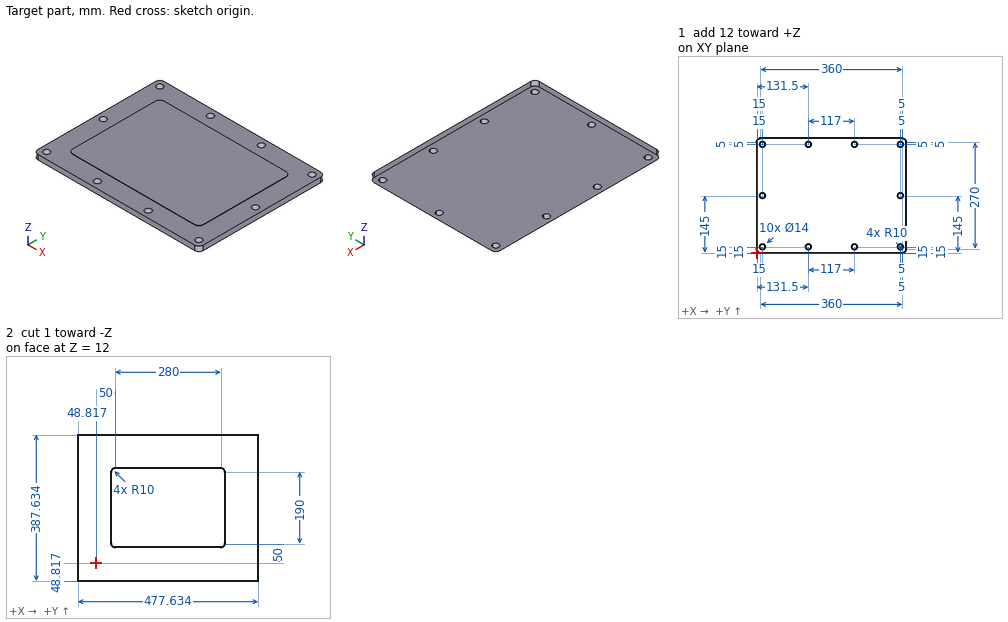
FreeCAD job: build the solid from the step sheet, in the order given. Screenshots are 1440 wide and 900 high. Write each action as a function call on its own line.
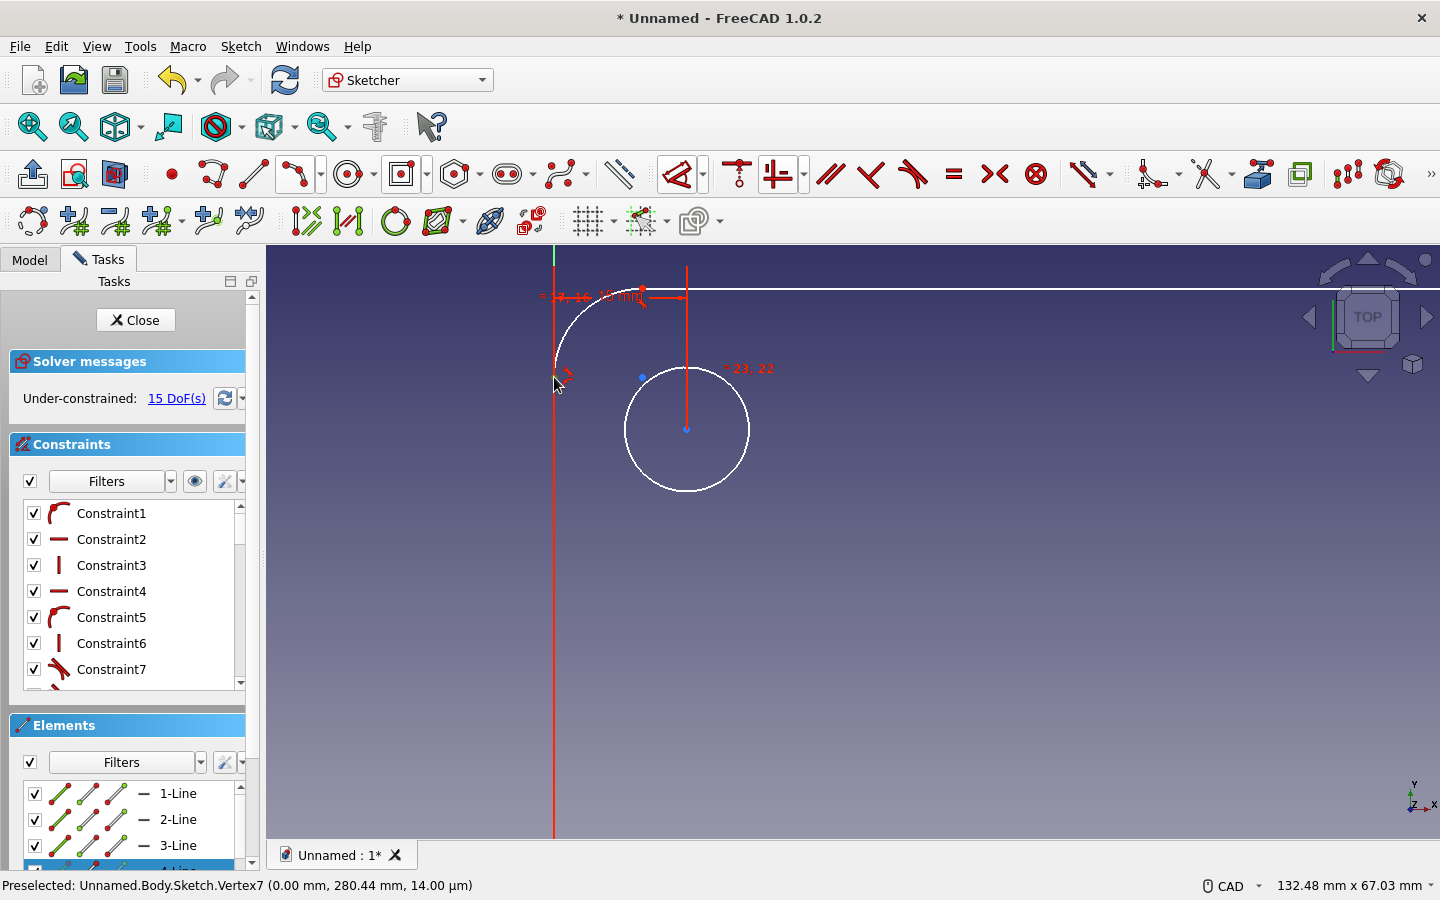
click(687, 429)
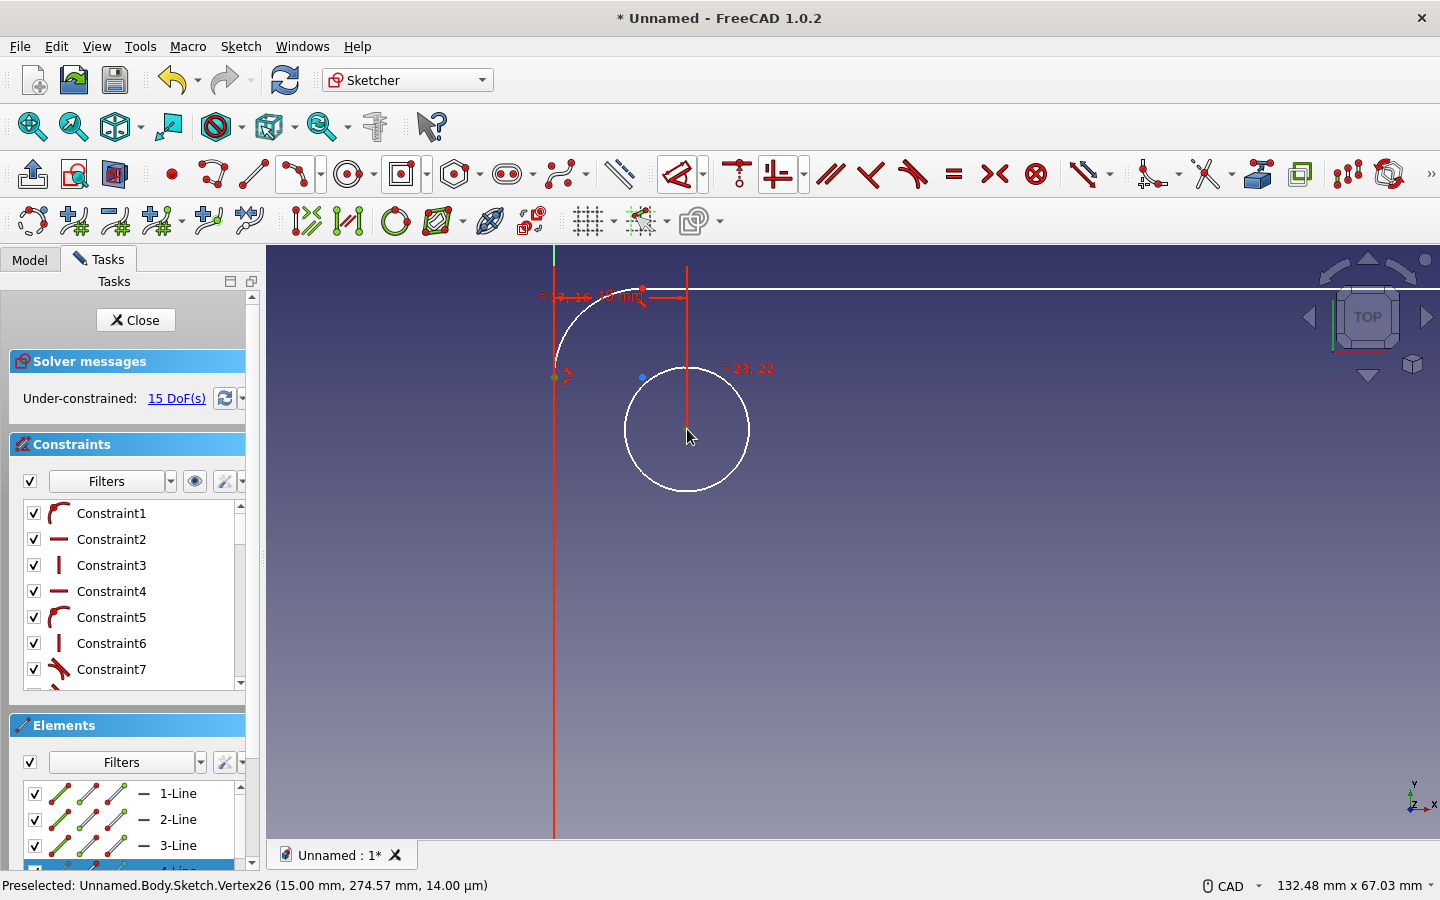
key(i)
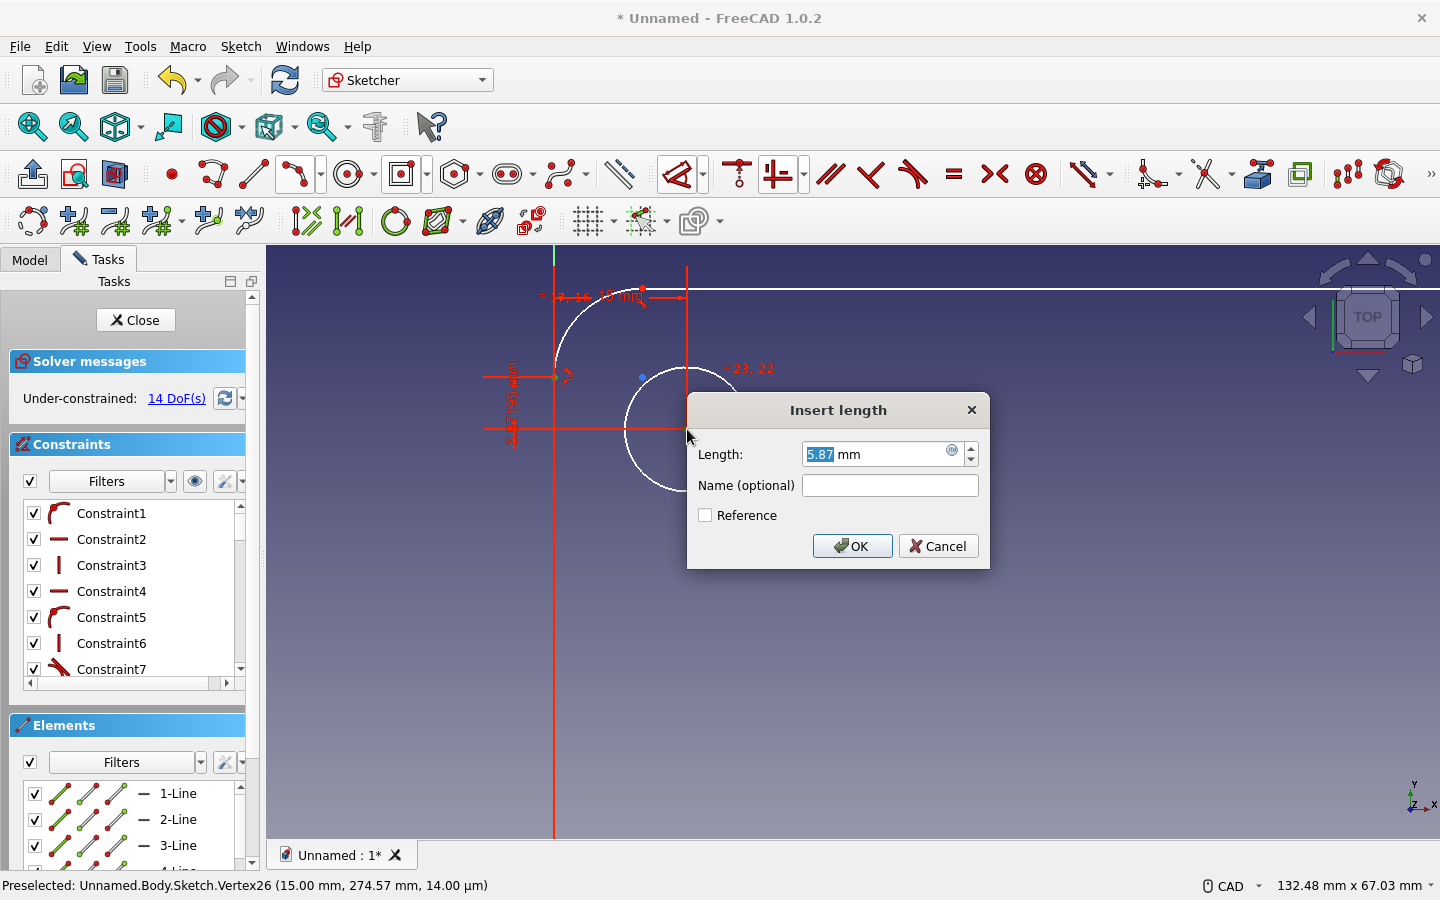
text(5)
key(Return)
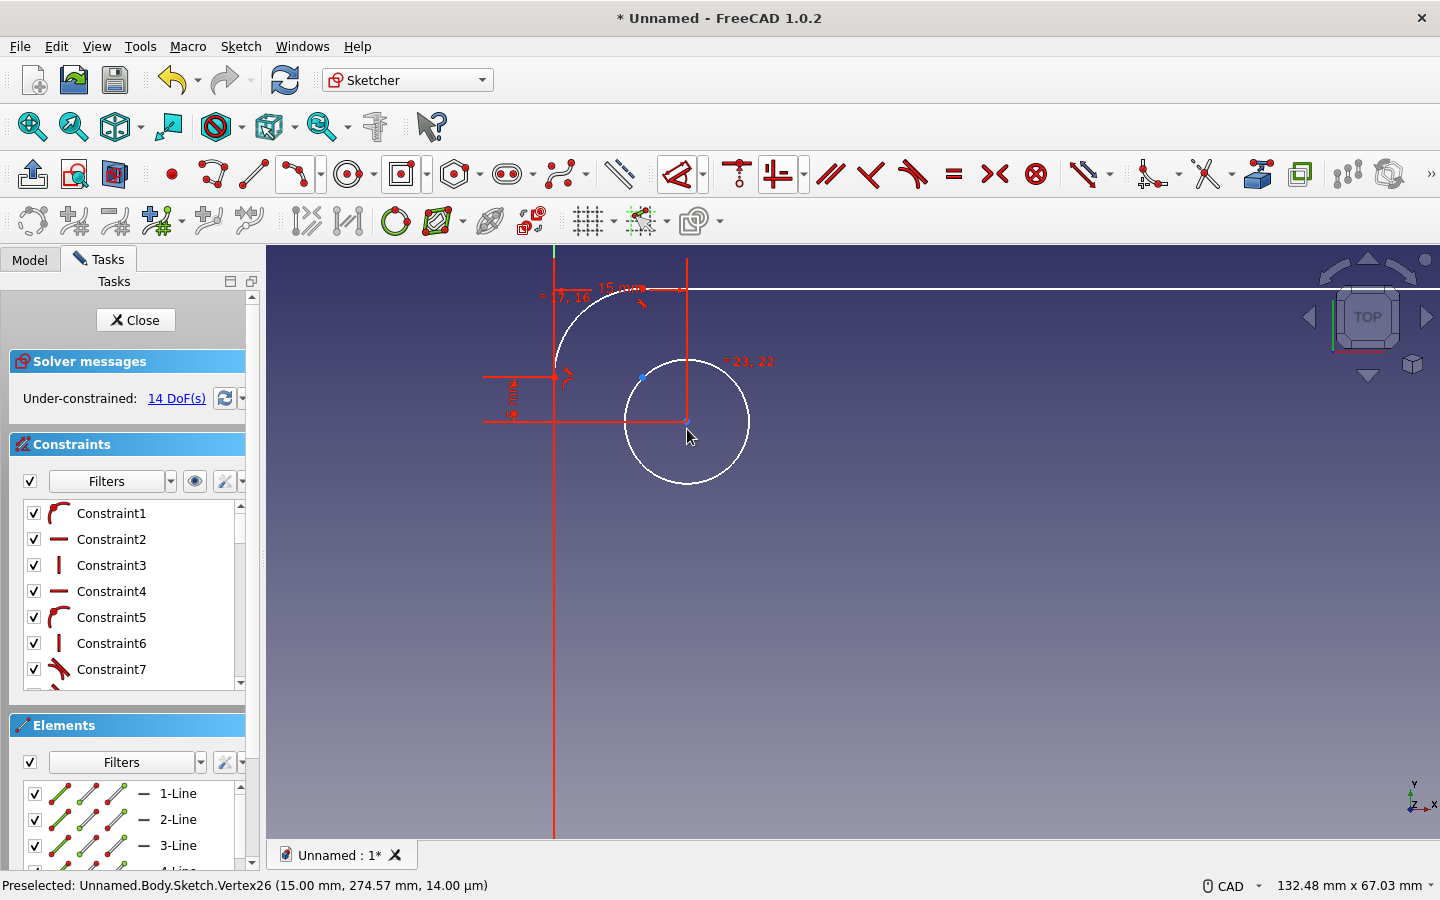
click(554, 377)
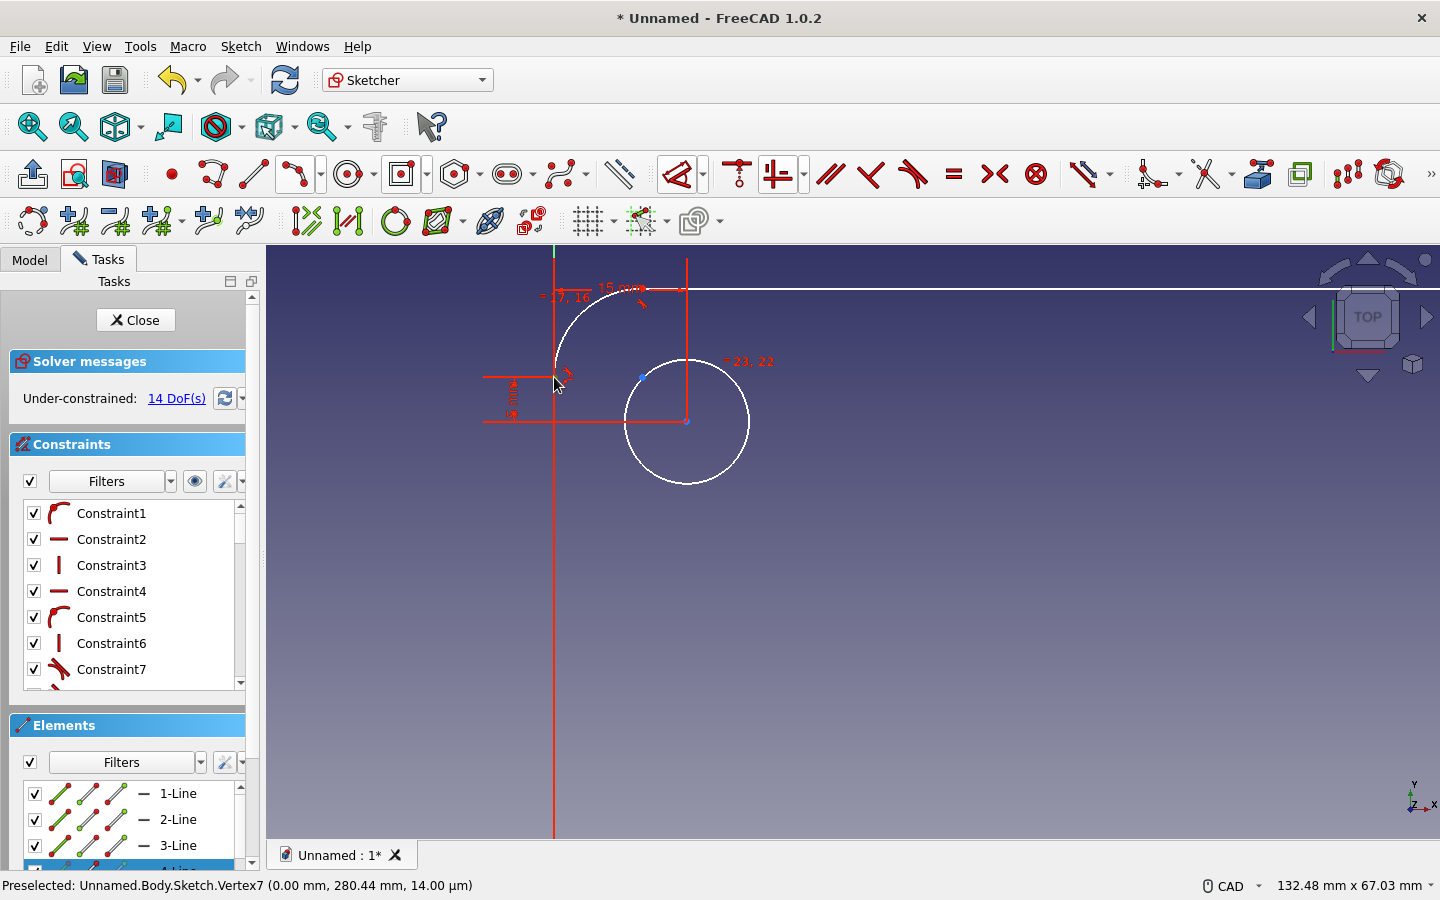
scroll(557, 380, down, 10)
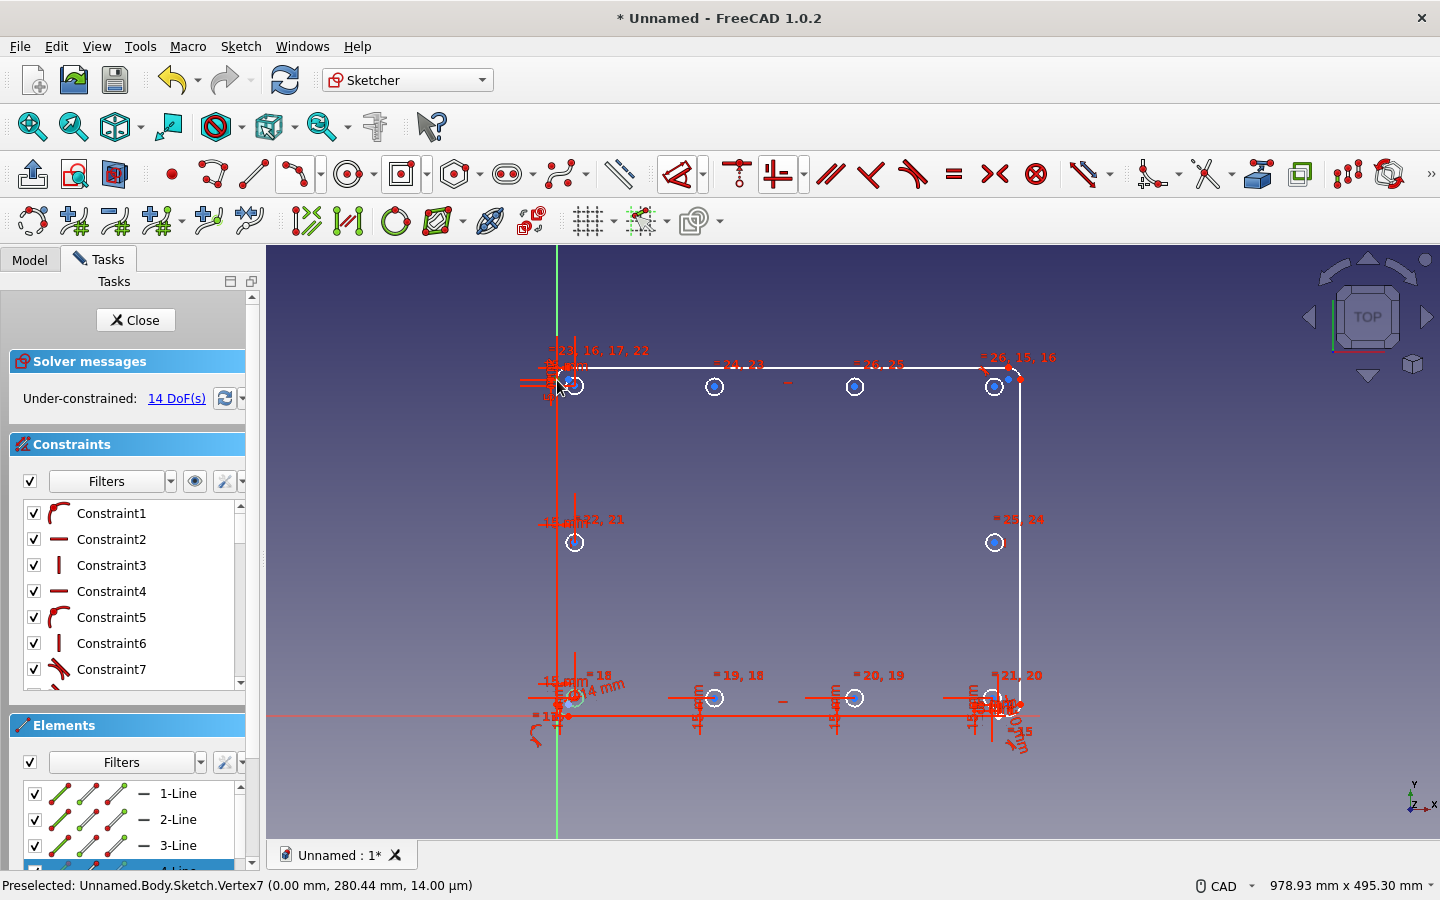
scroll(715, 387, up, 10)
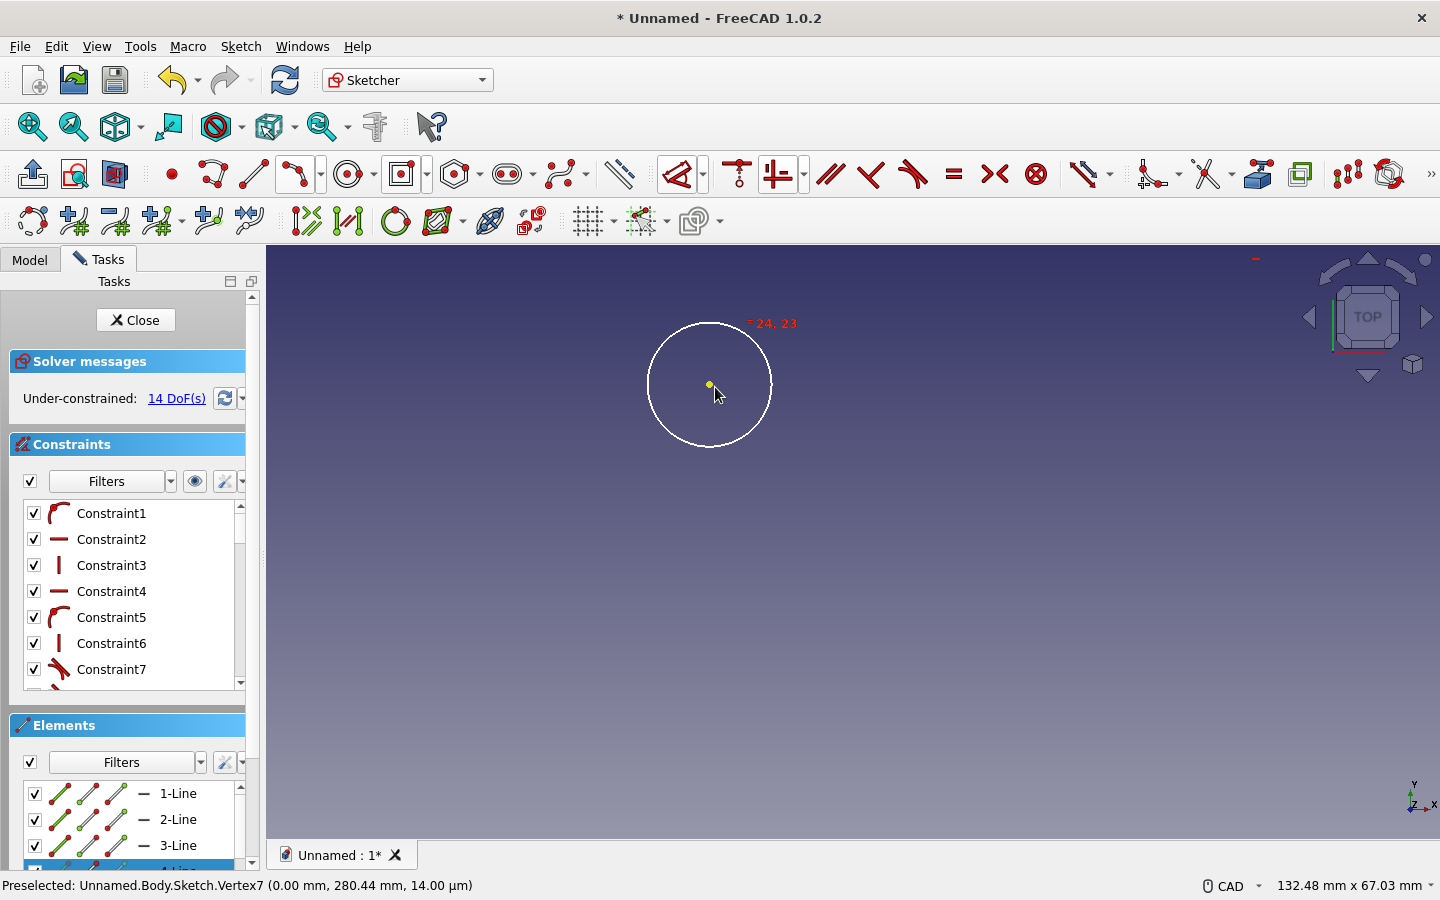
click(710, 385)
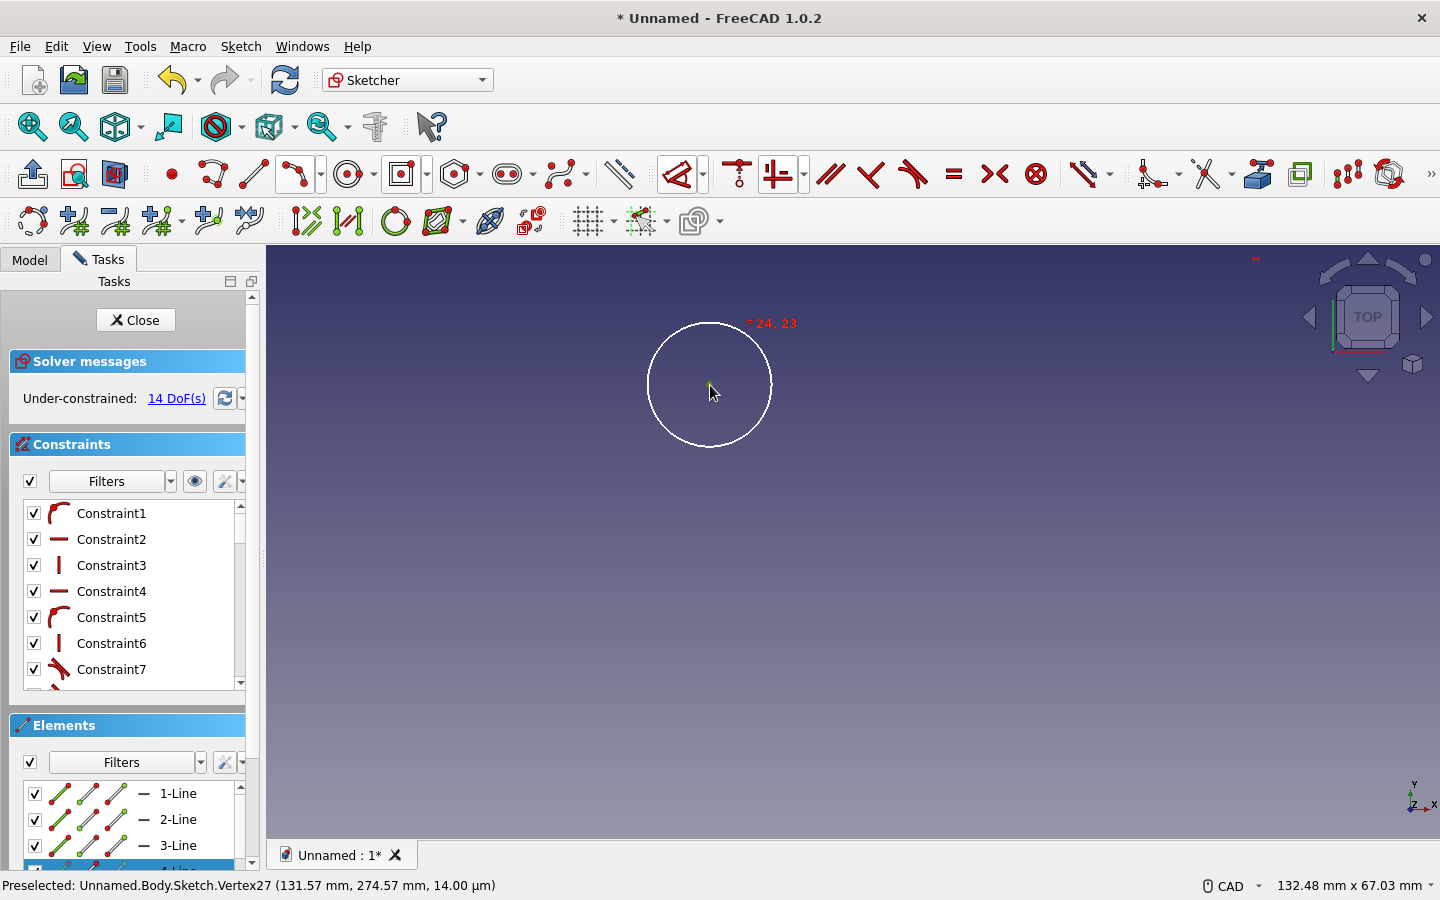
key(i)